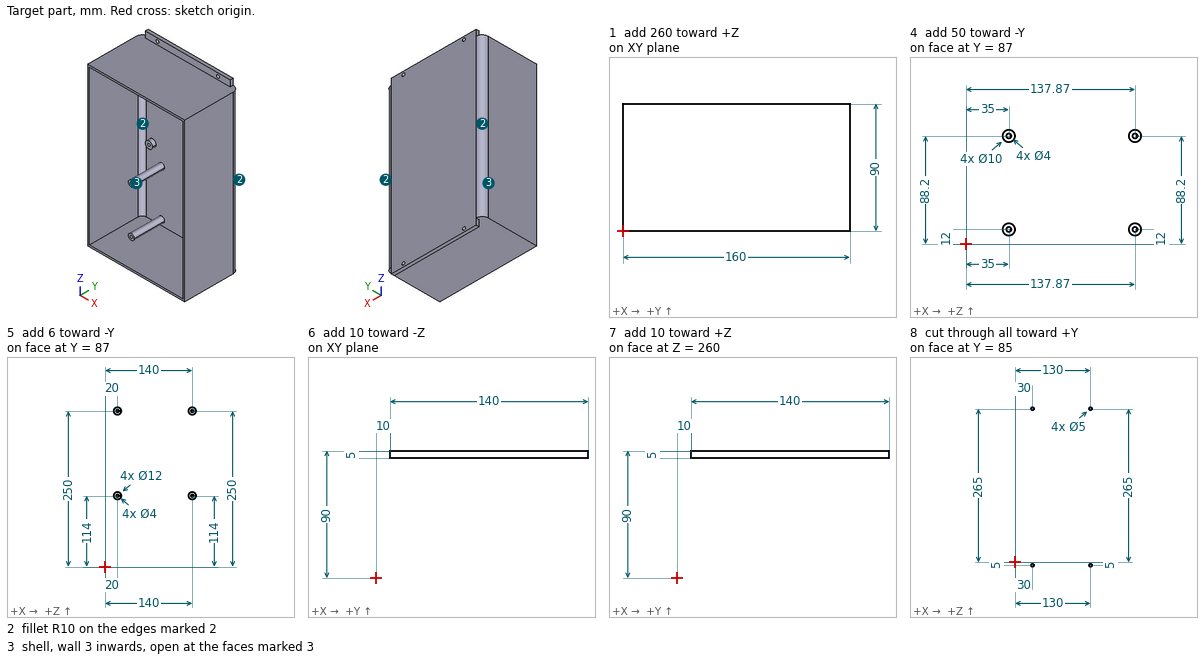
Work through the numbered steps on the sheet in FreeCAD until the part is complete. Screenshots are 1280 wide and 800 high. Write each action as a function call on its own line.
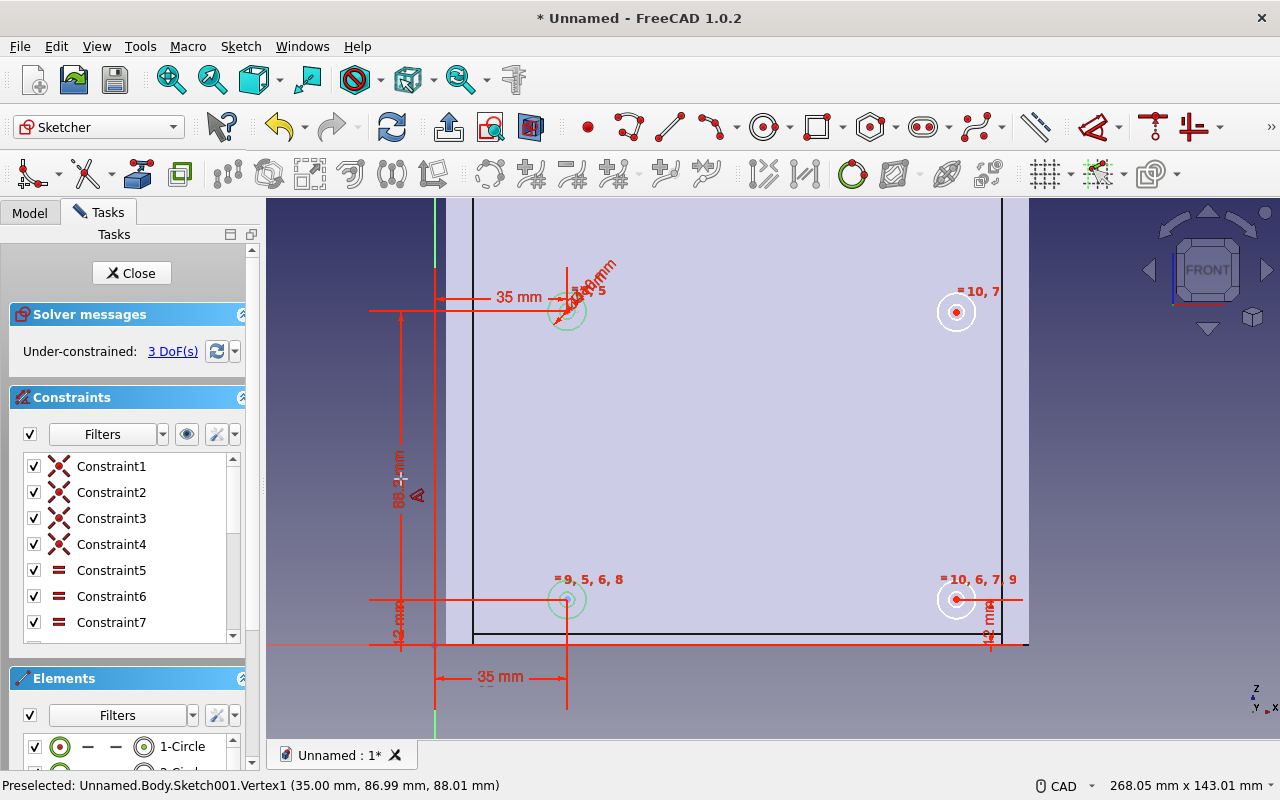
click(957, 312)
click(401, 402)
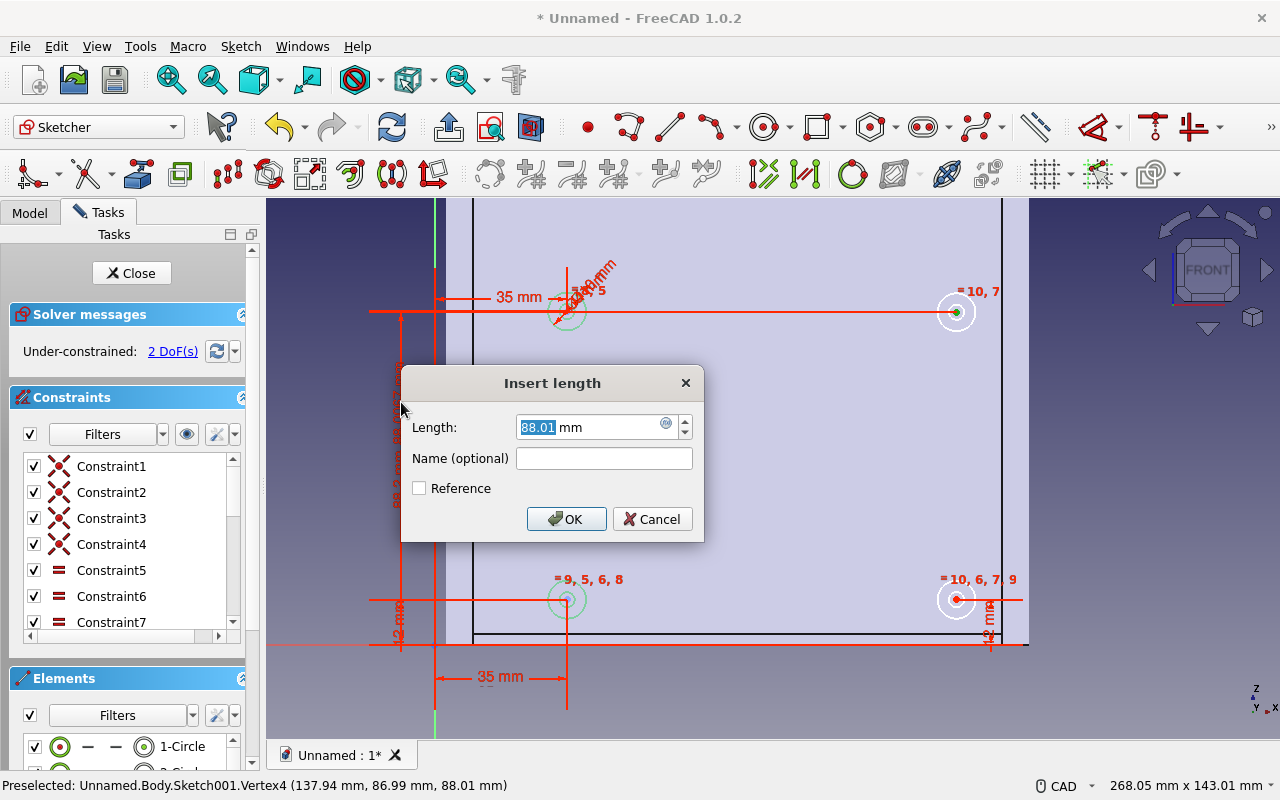
text(88.2)
key(Return)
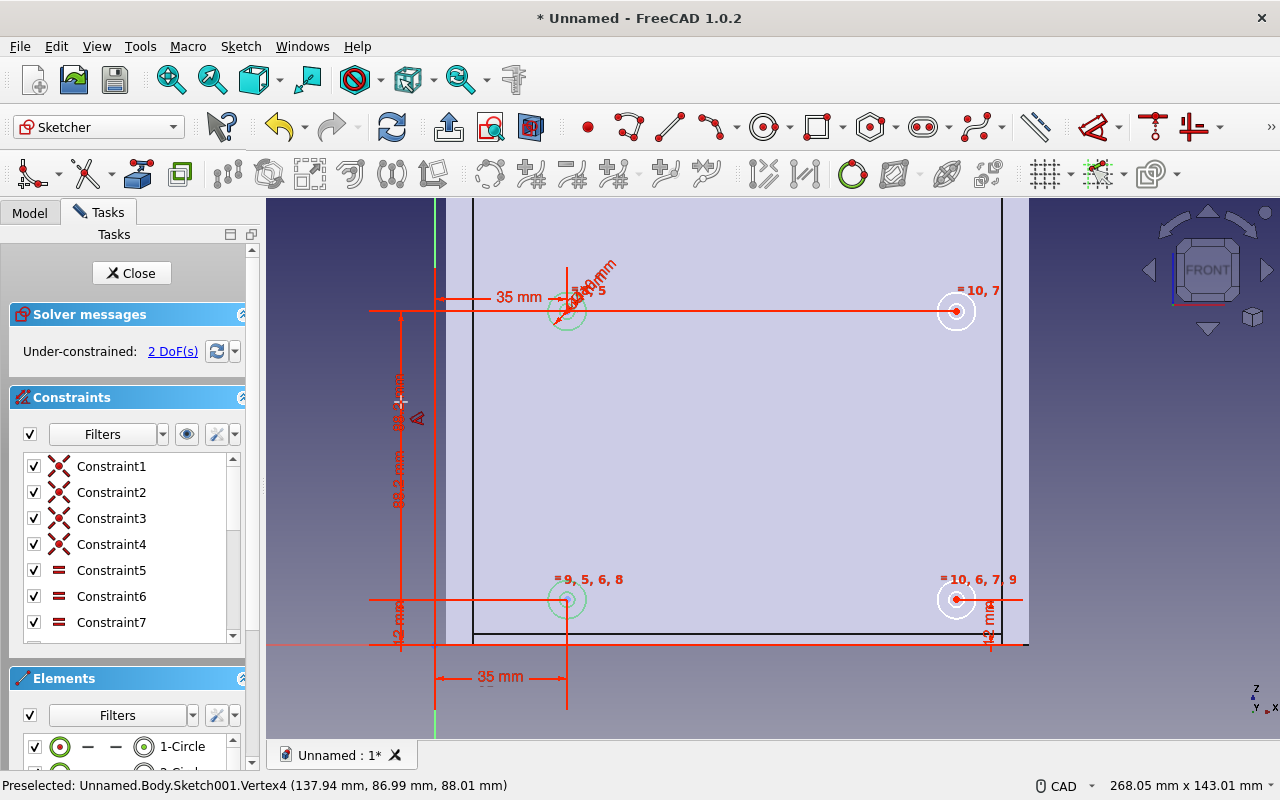
click(957, 600)
click(696, 679)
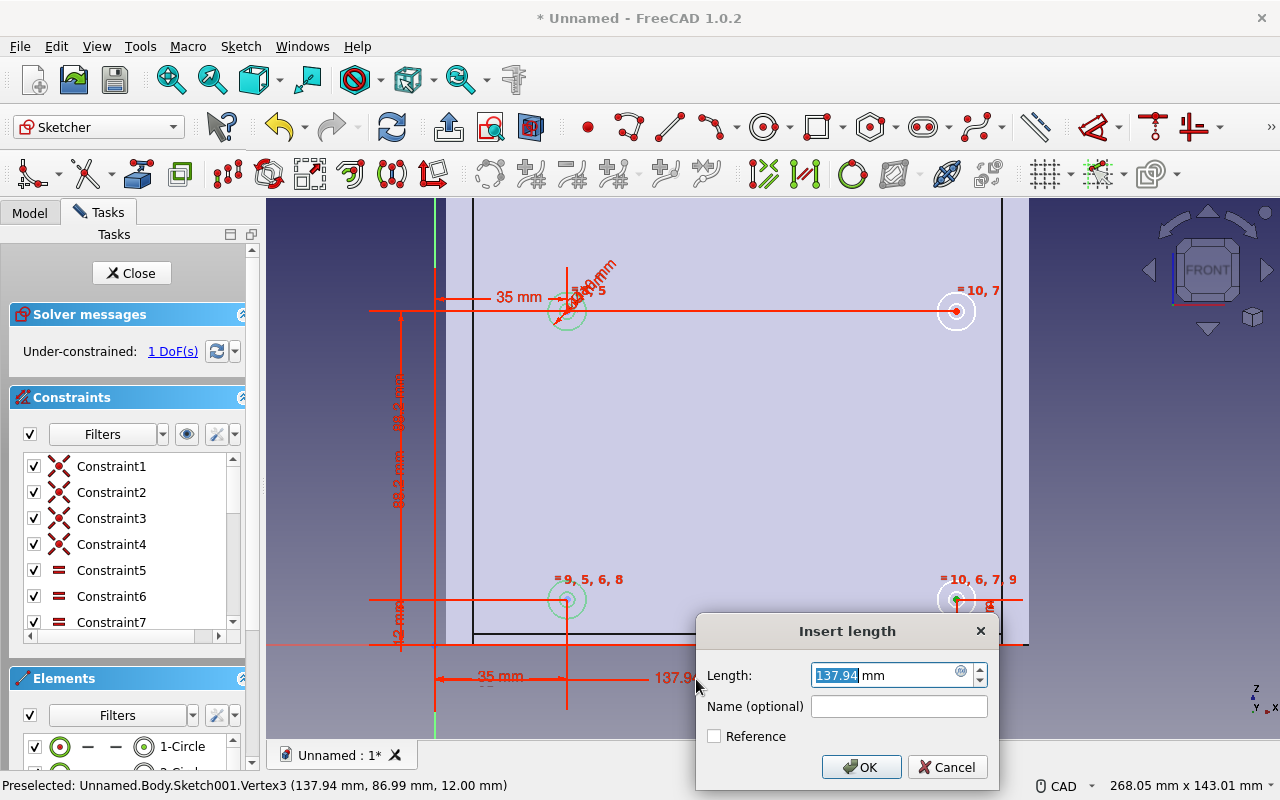
text(137.87)
key(Return)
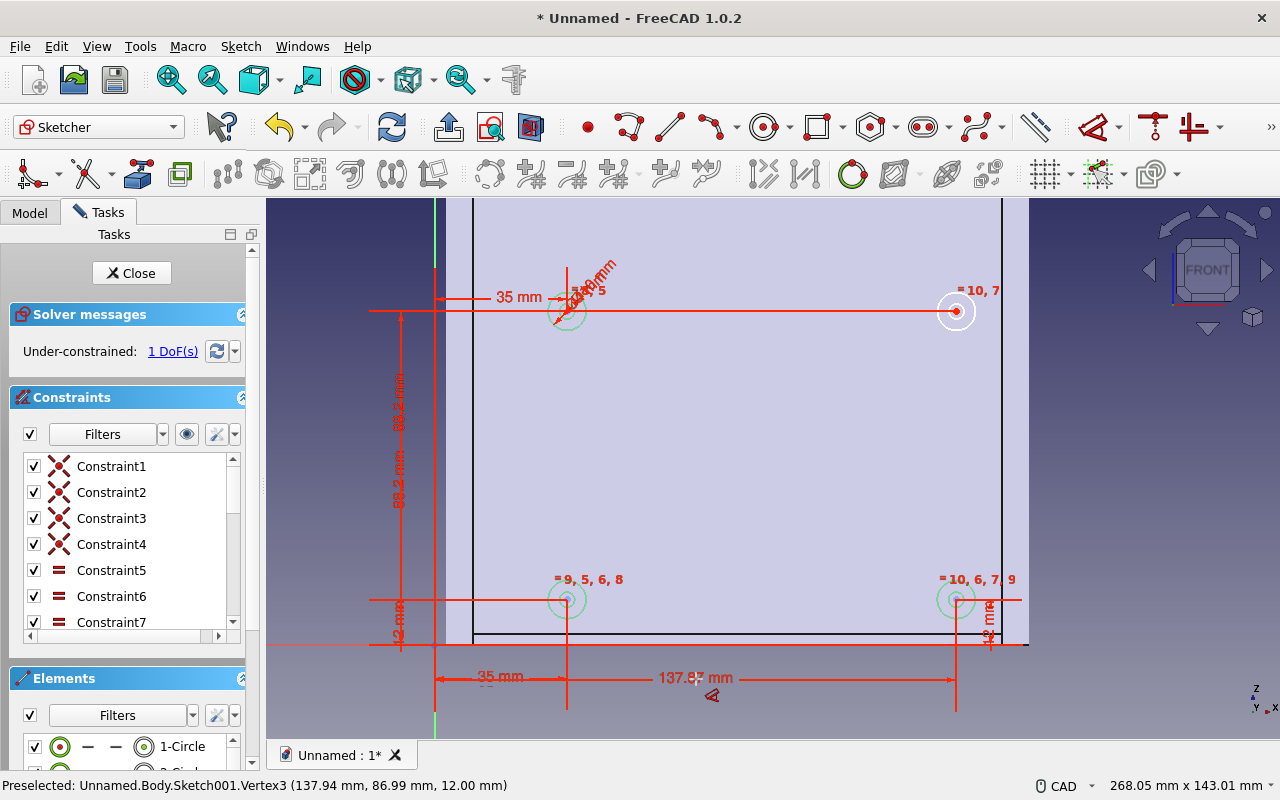
click(957, 311)
click(576, 679)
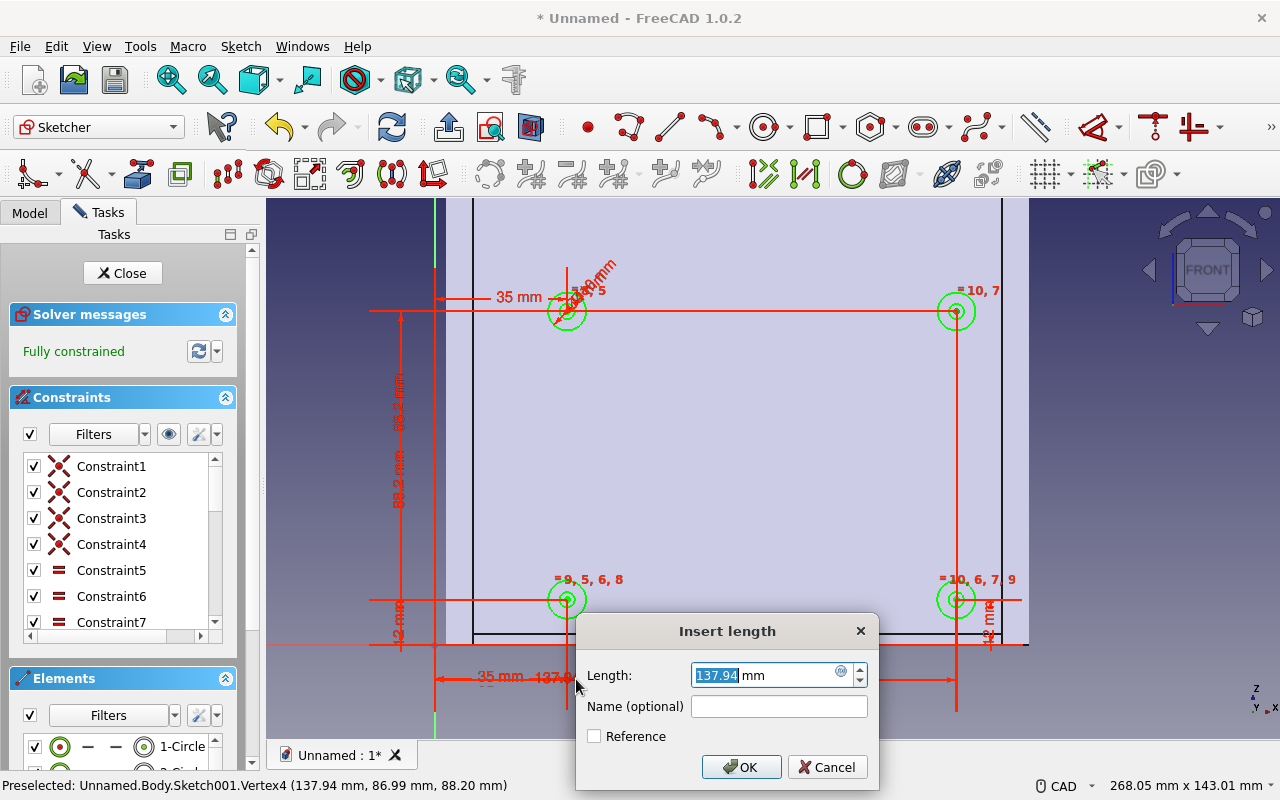
text(137.87)
key(Return)
key(Escape)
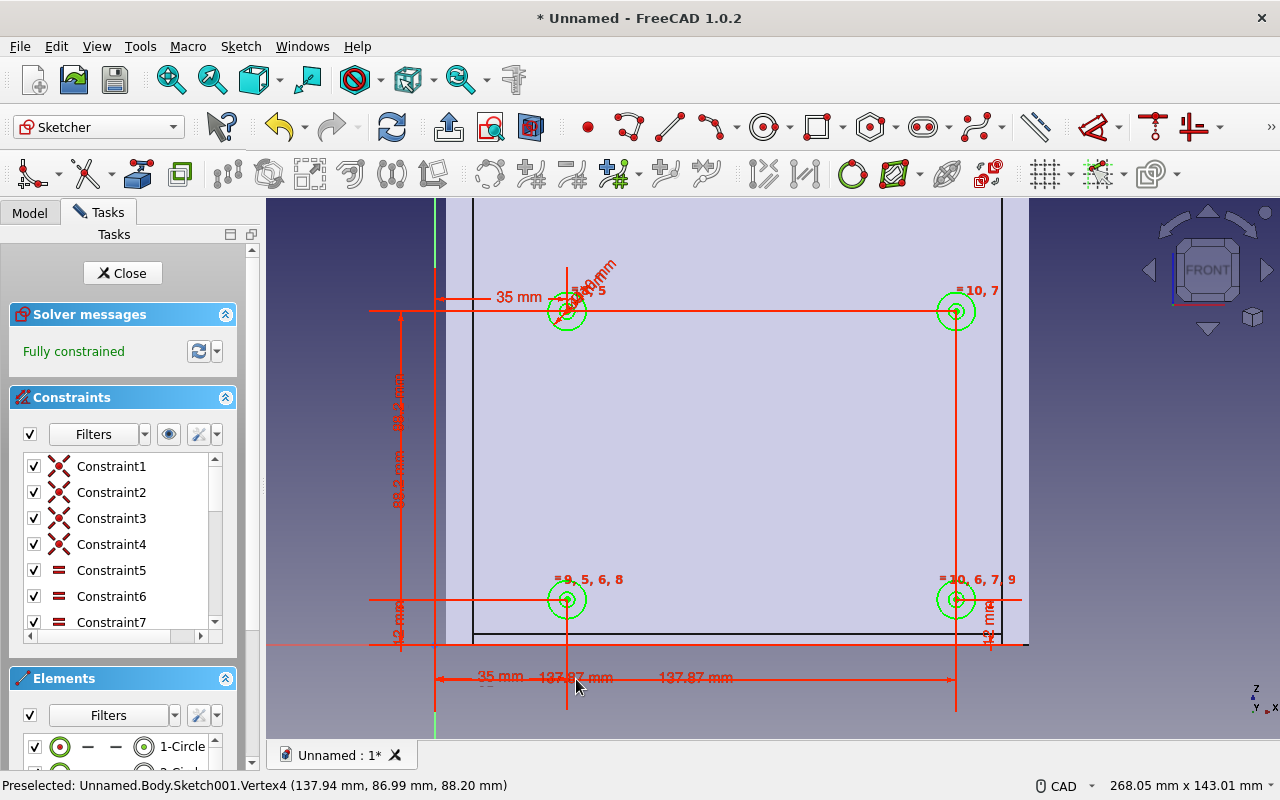
click(123, 273)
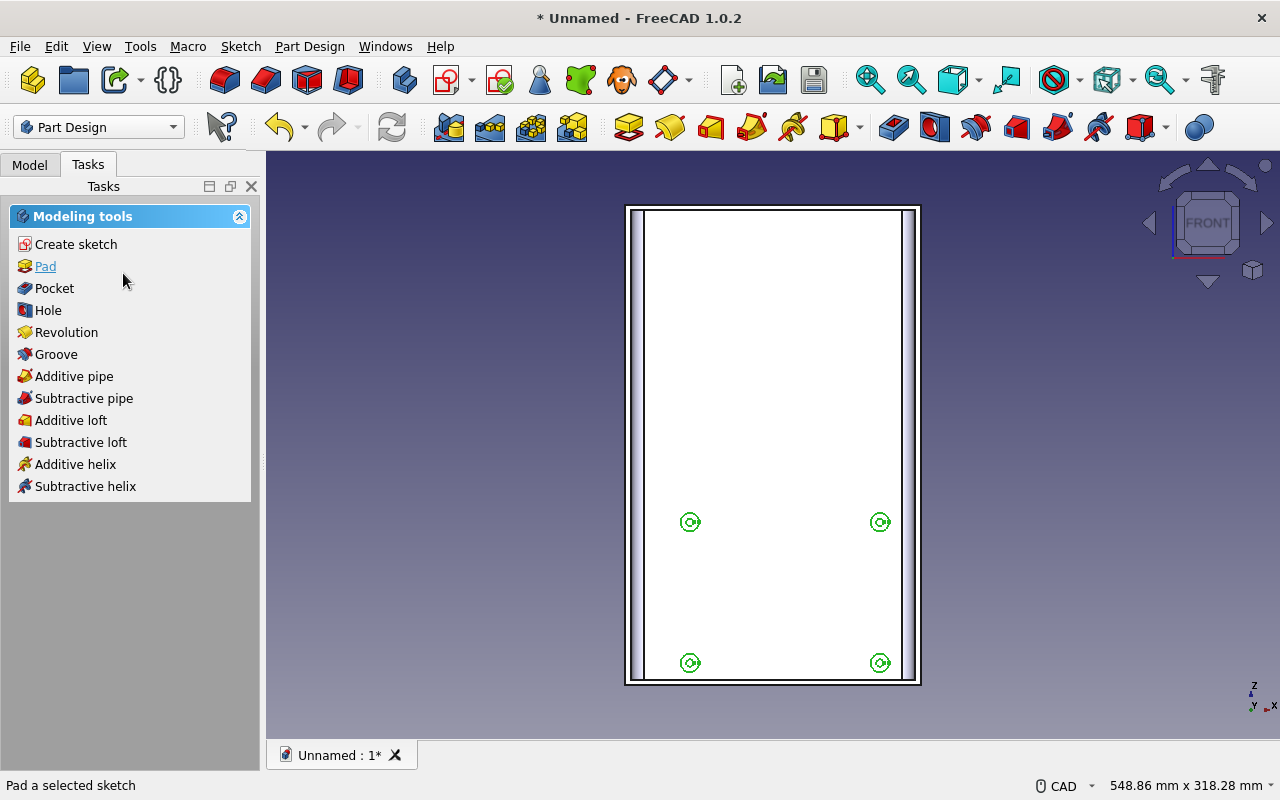
click(629, 128)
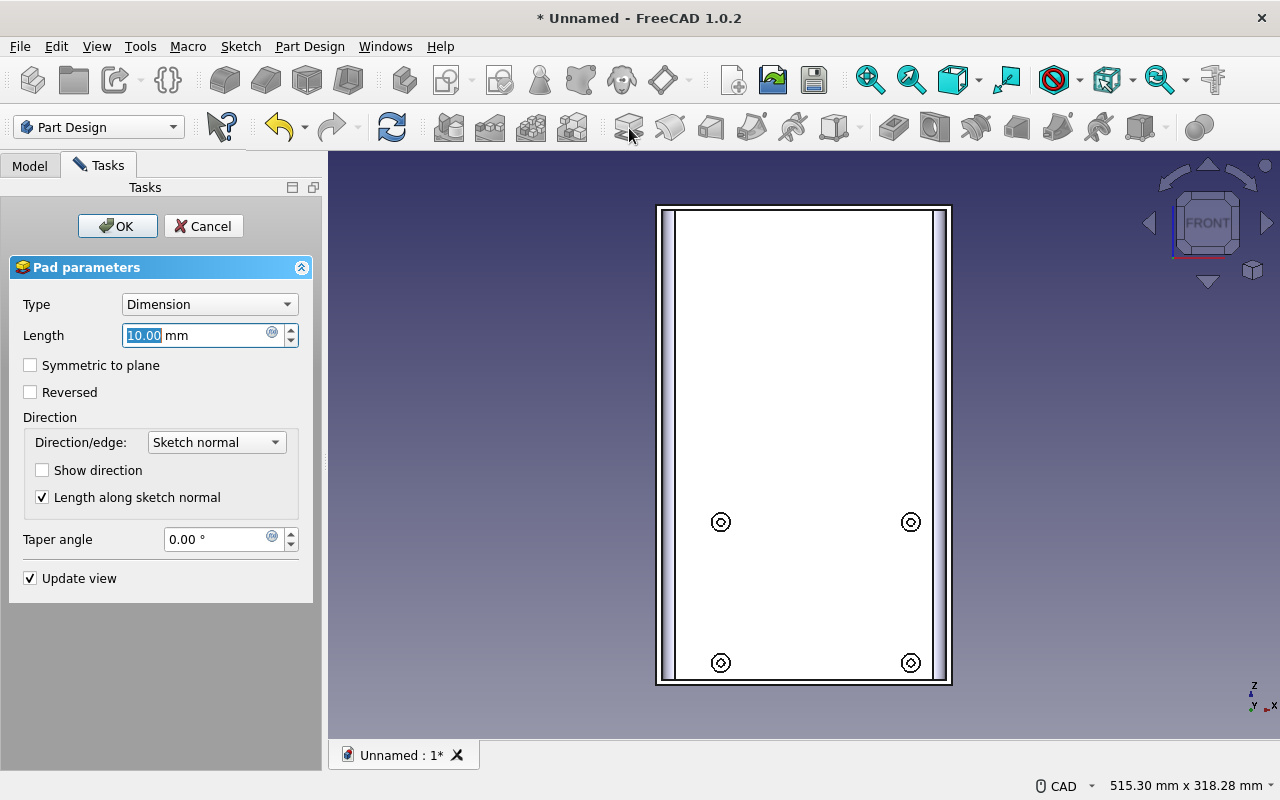
text(50)
key(Tab)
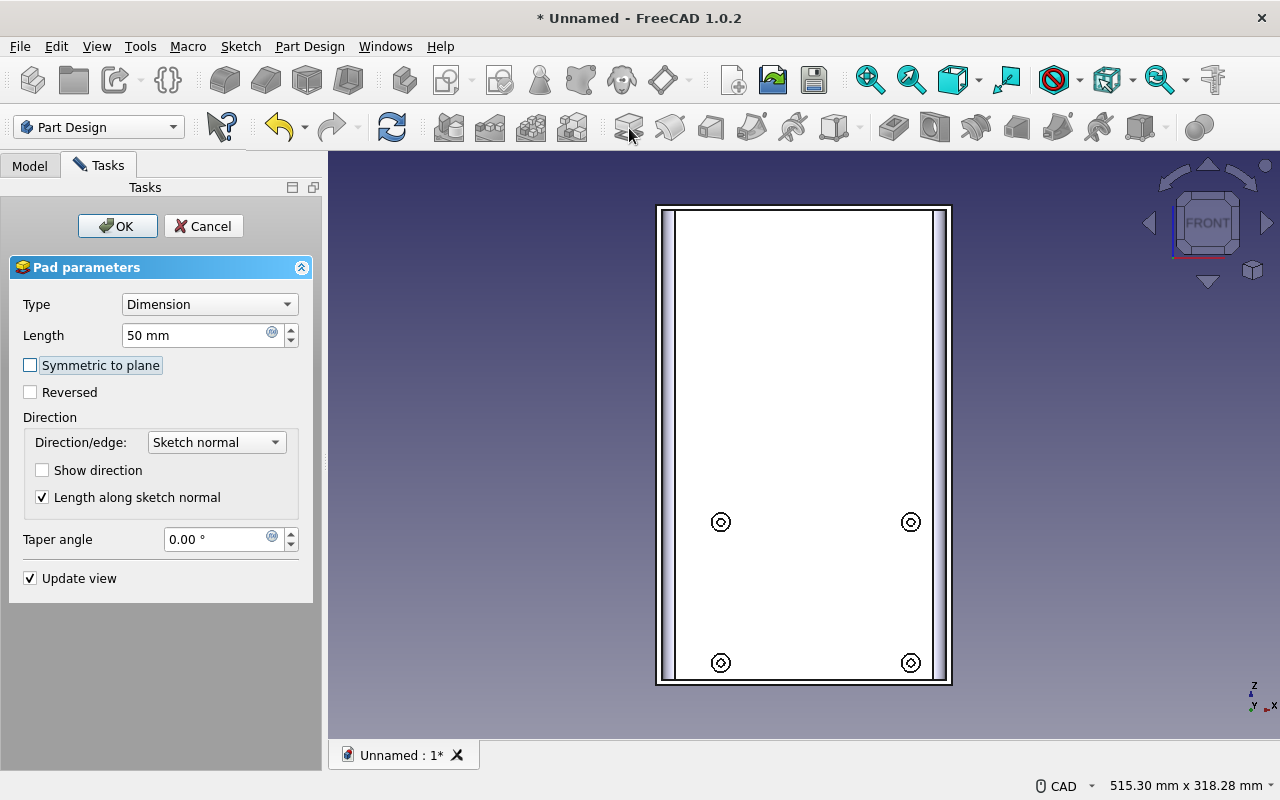
click(118, 226)